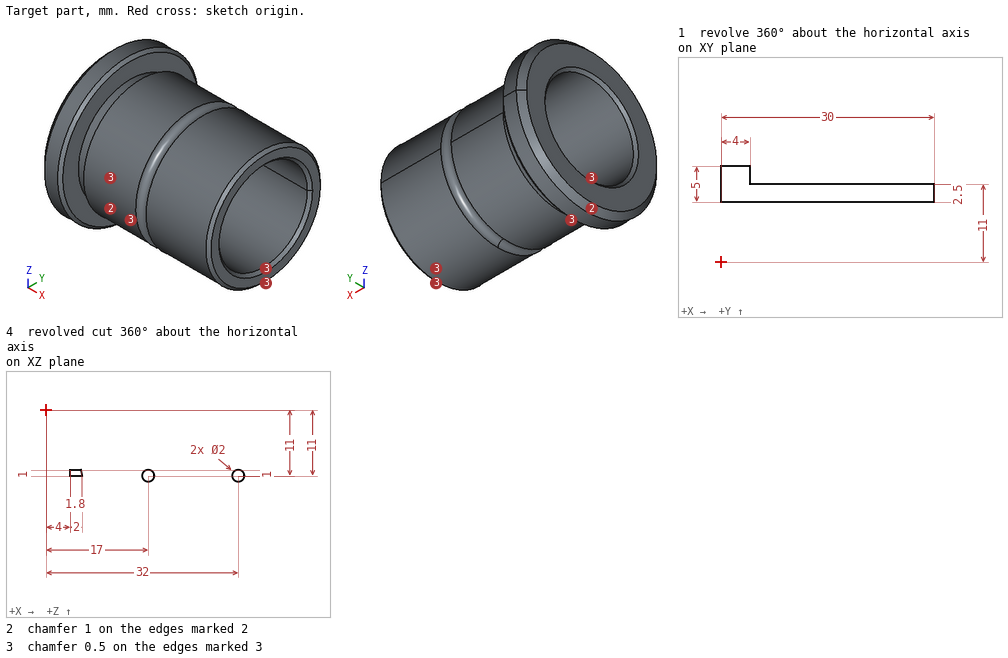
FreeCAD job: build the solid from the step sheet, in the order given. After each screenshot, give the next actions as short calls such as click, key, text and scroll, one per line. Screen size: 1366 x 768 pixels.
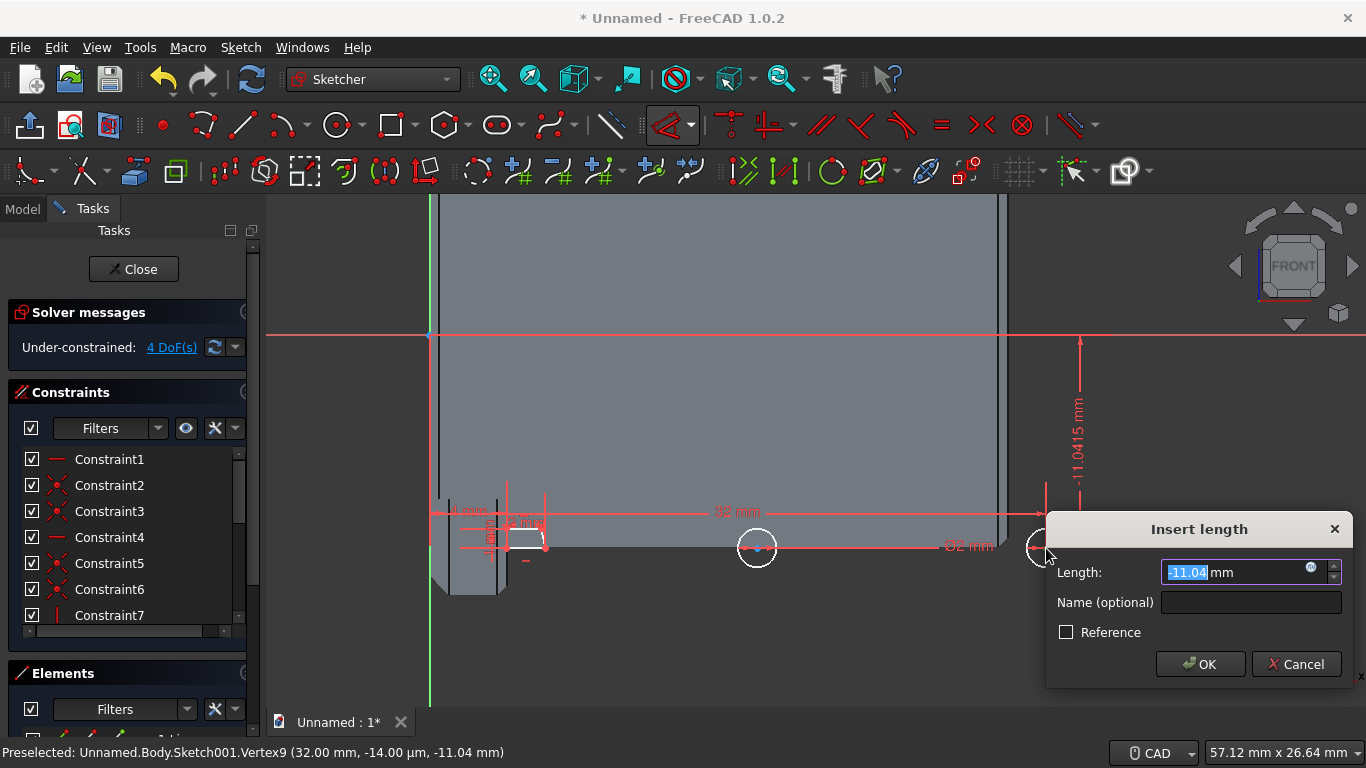
text(-11)
key(Return)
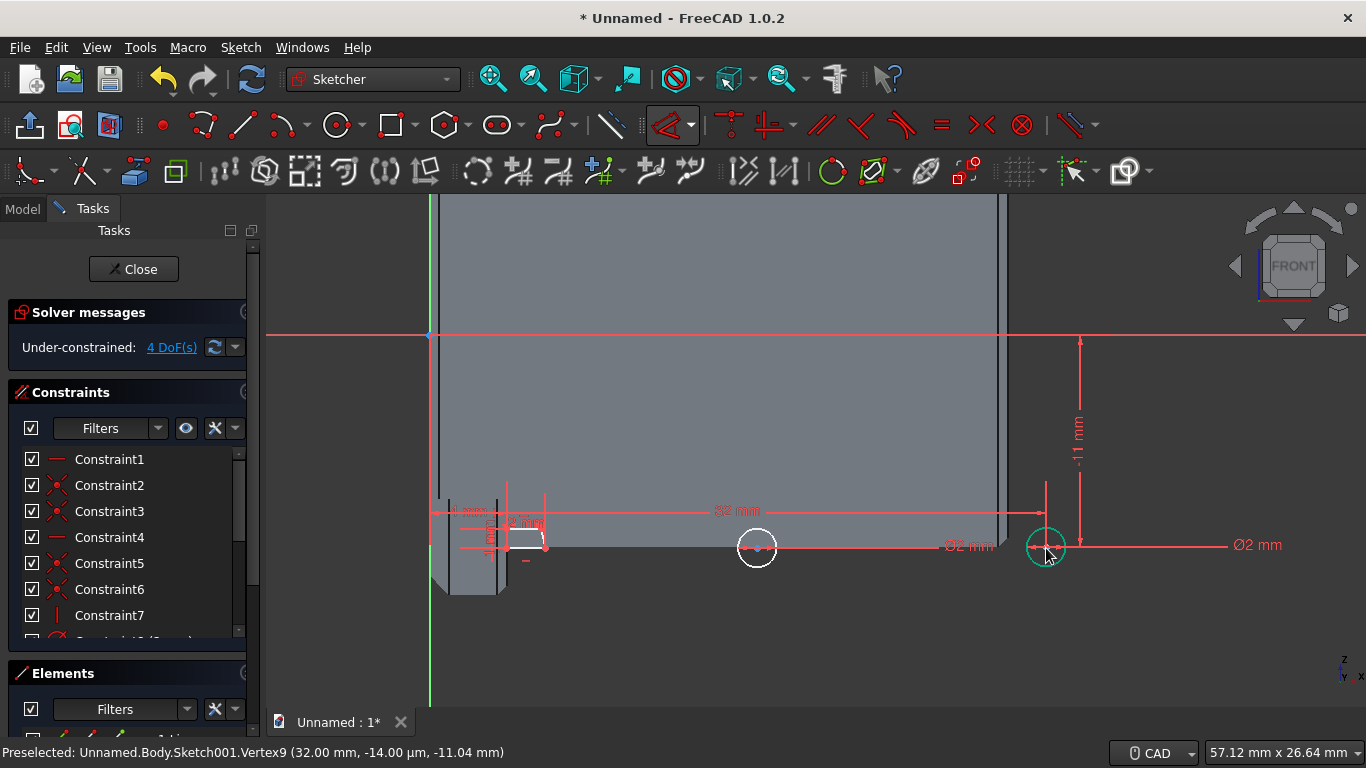
click(757, 548)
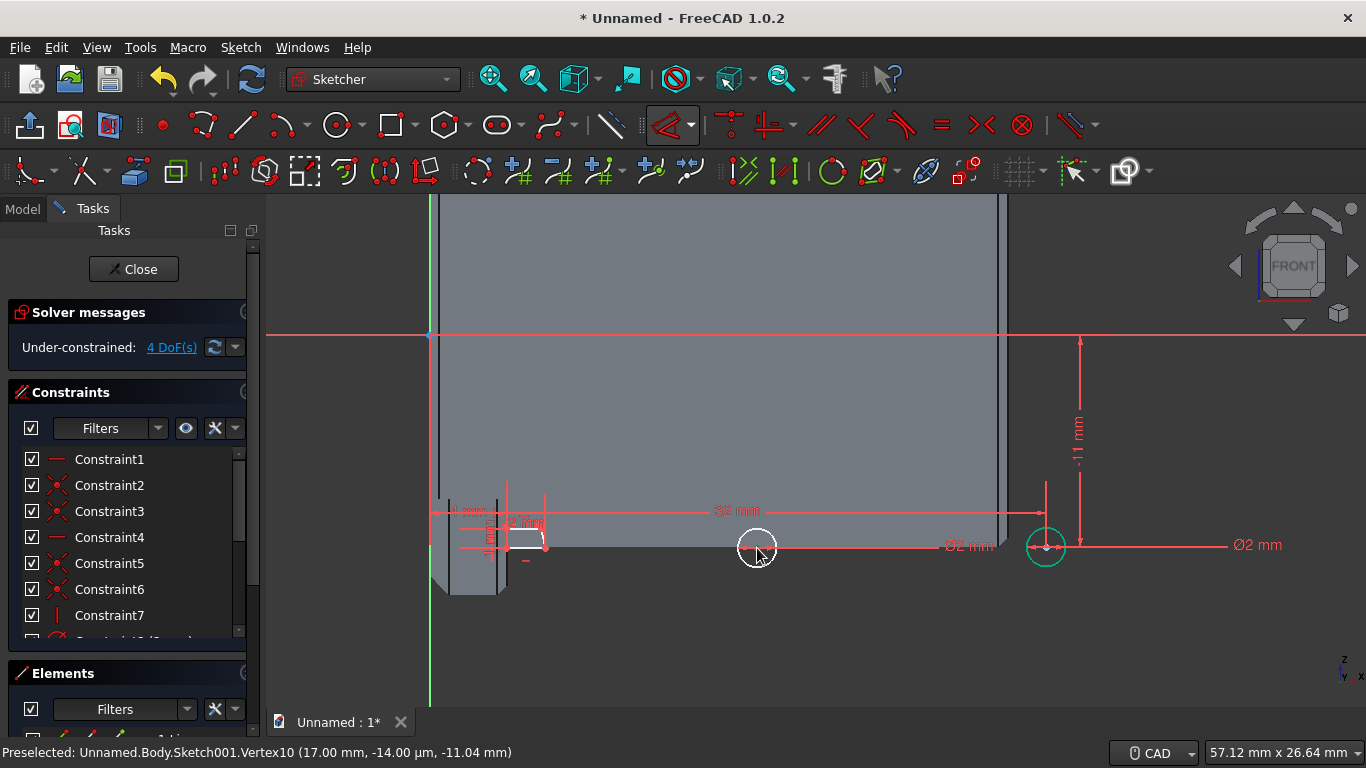
click(694, 126)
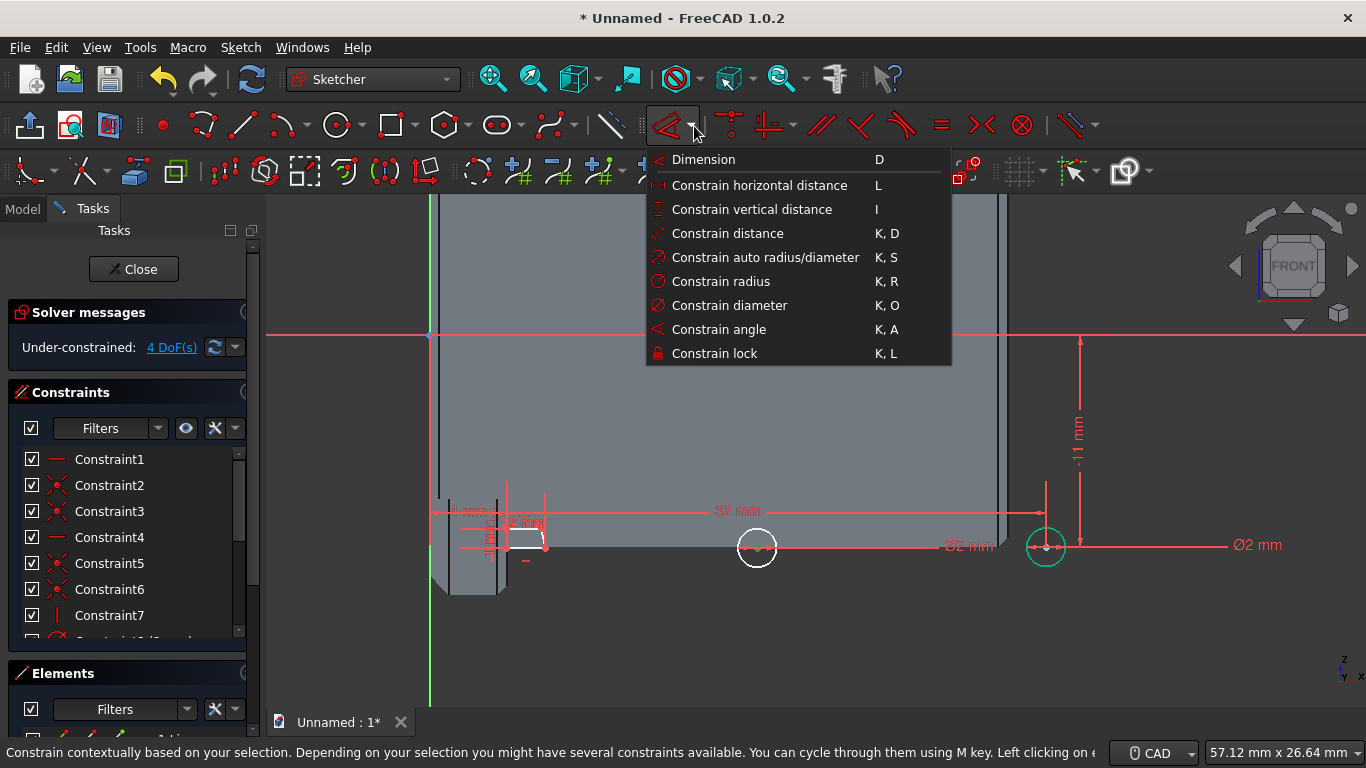
click(799, 185)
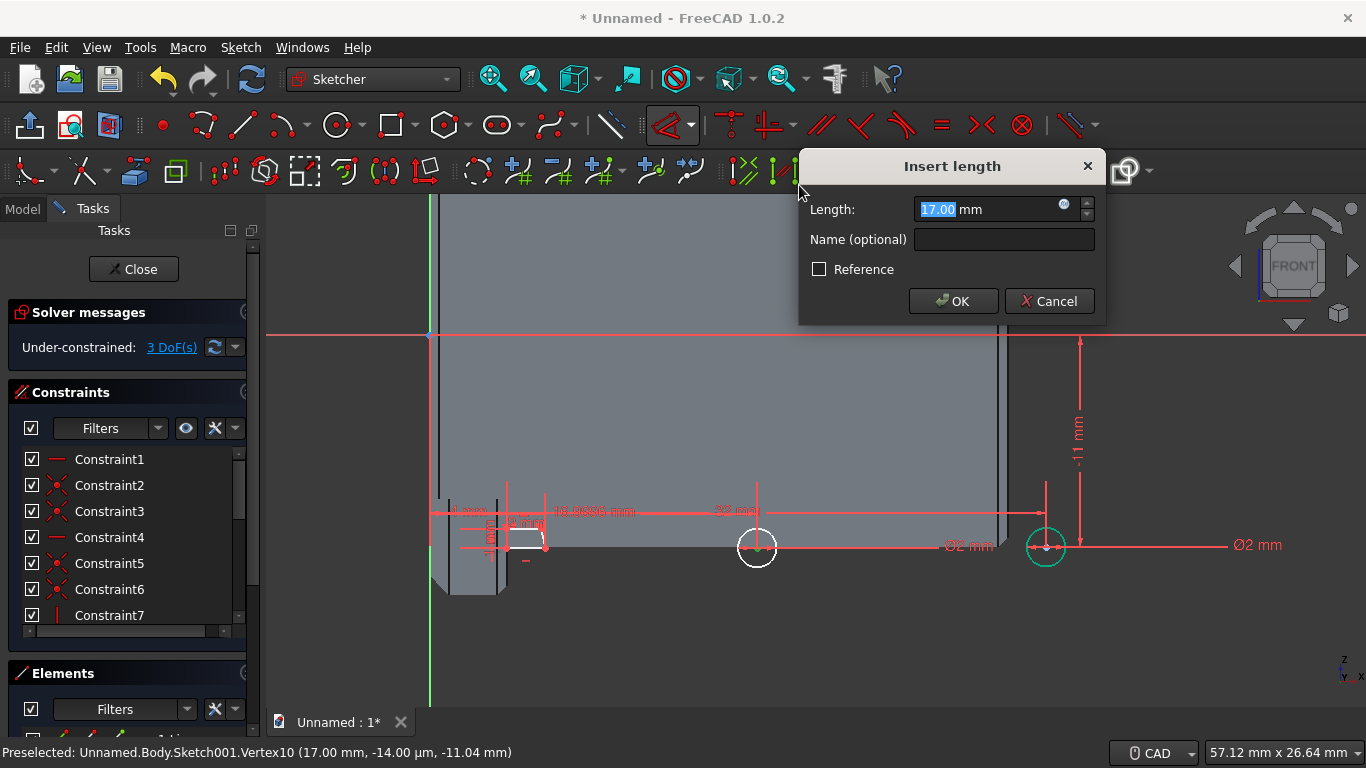
text(17)
key(Return)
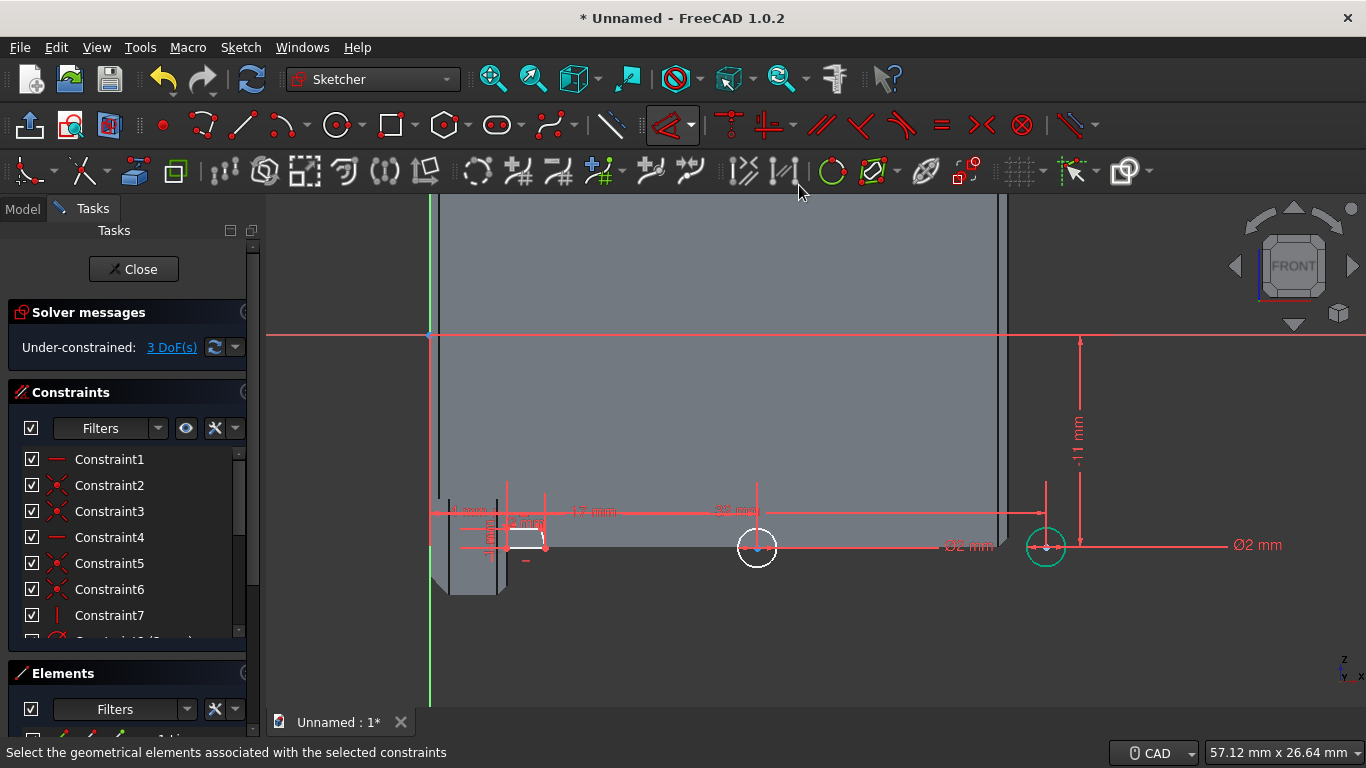
click(757, 548)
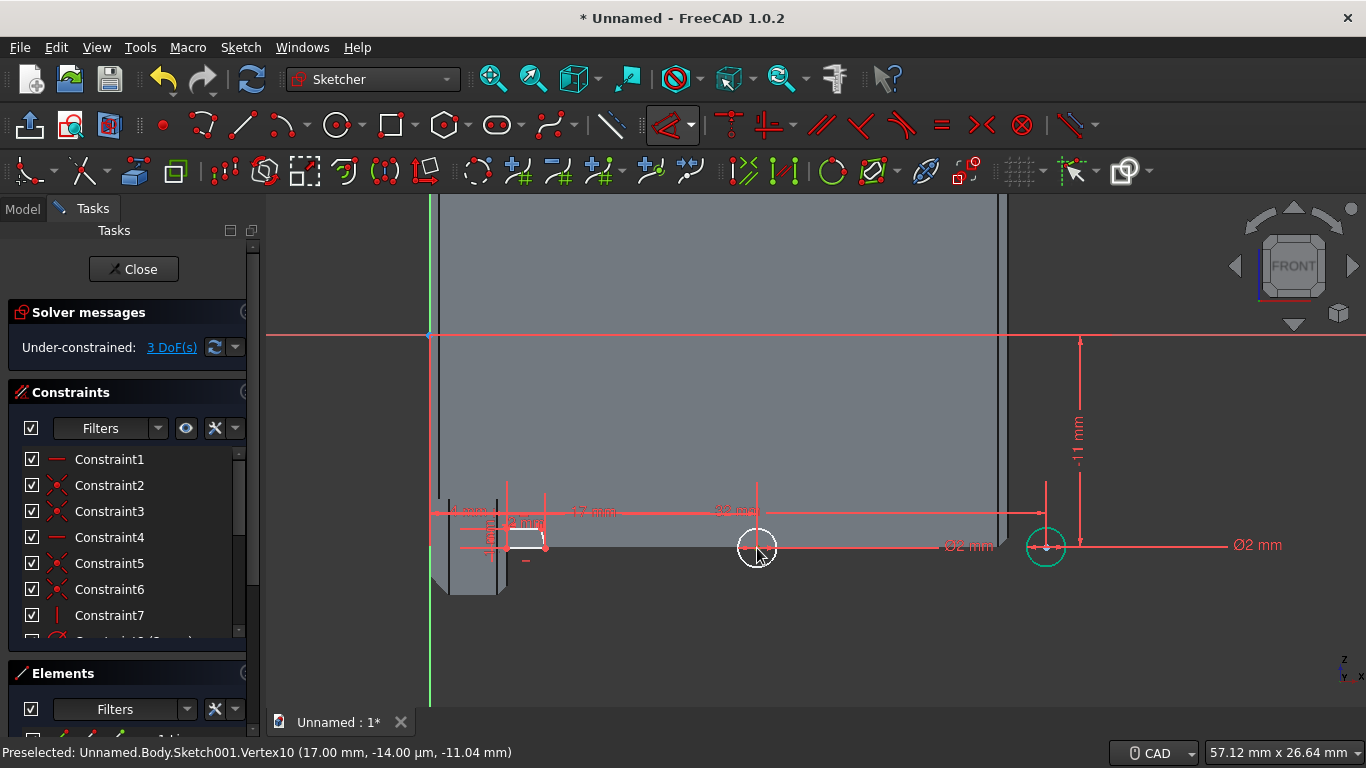
click(694, 126)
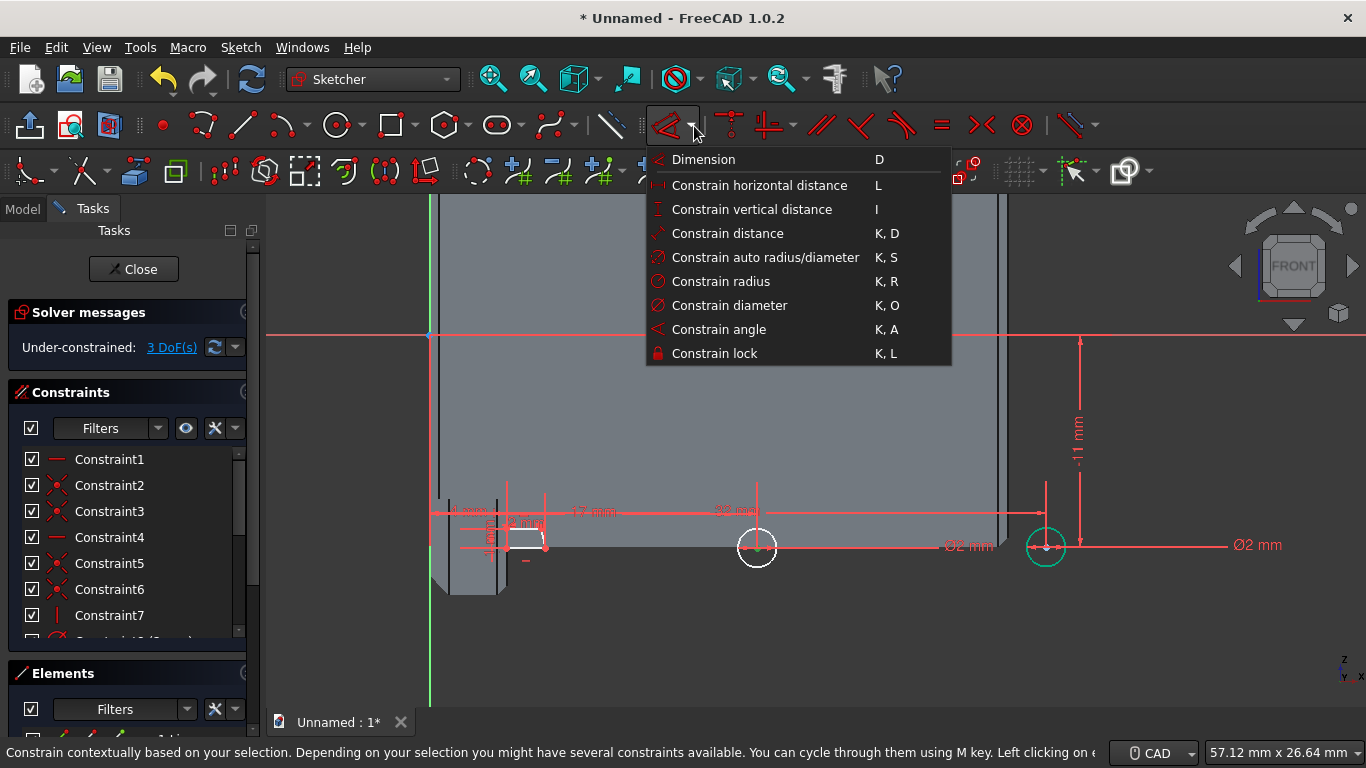
click(799, 209)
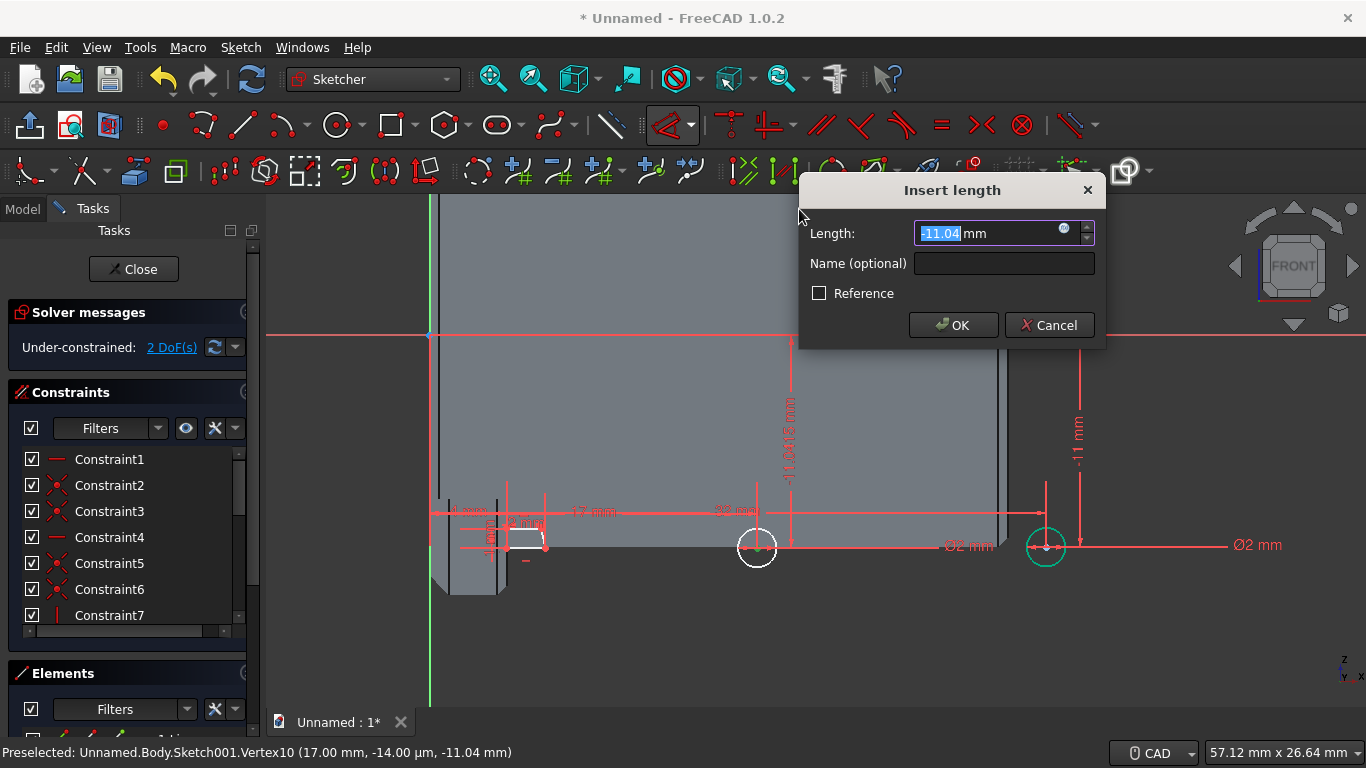
text(-11)
key(Return)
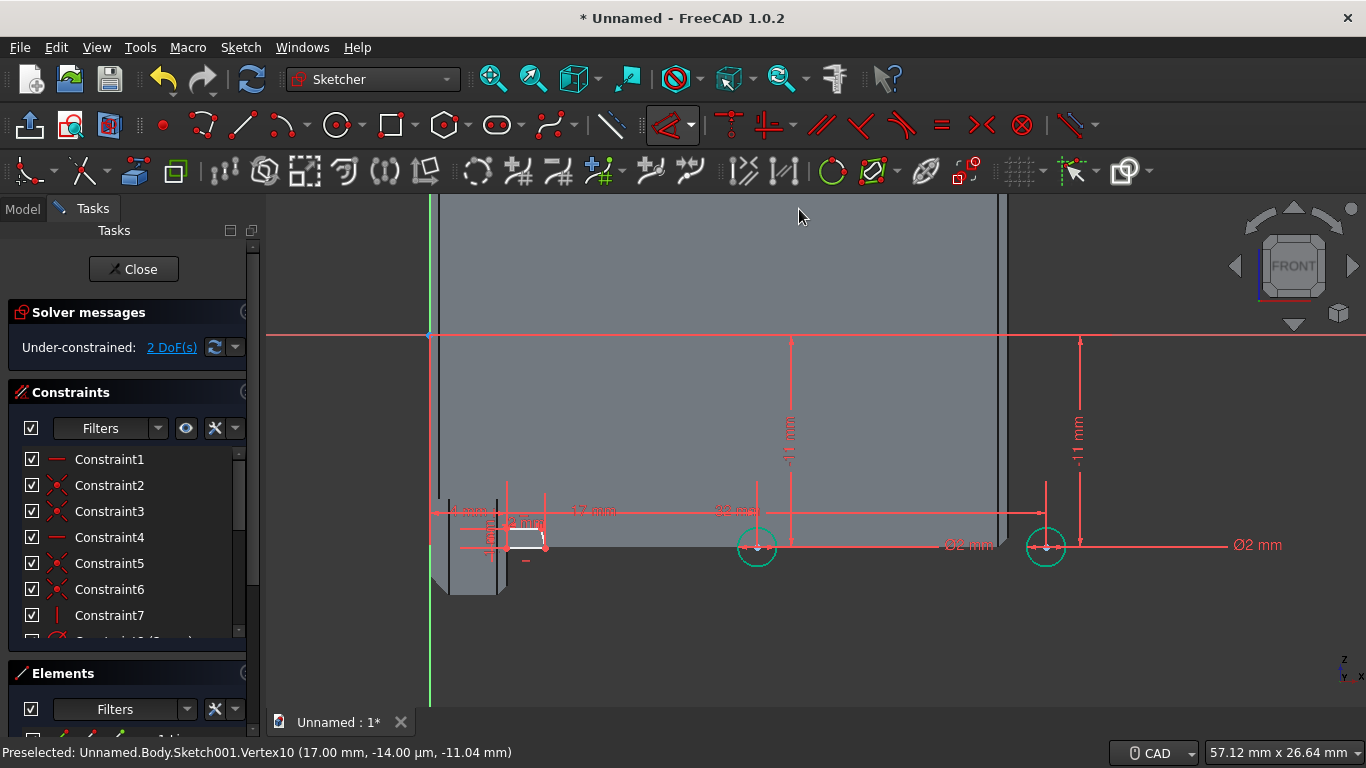
scroll(541, 529, up, 4)